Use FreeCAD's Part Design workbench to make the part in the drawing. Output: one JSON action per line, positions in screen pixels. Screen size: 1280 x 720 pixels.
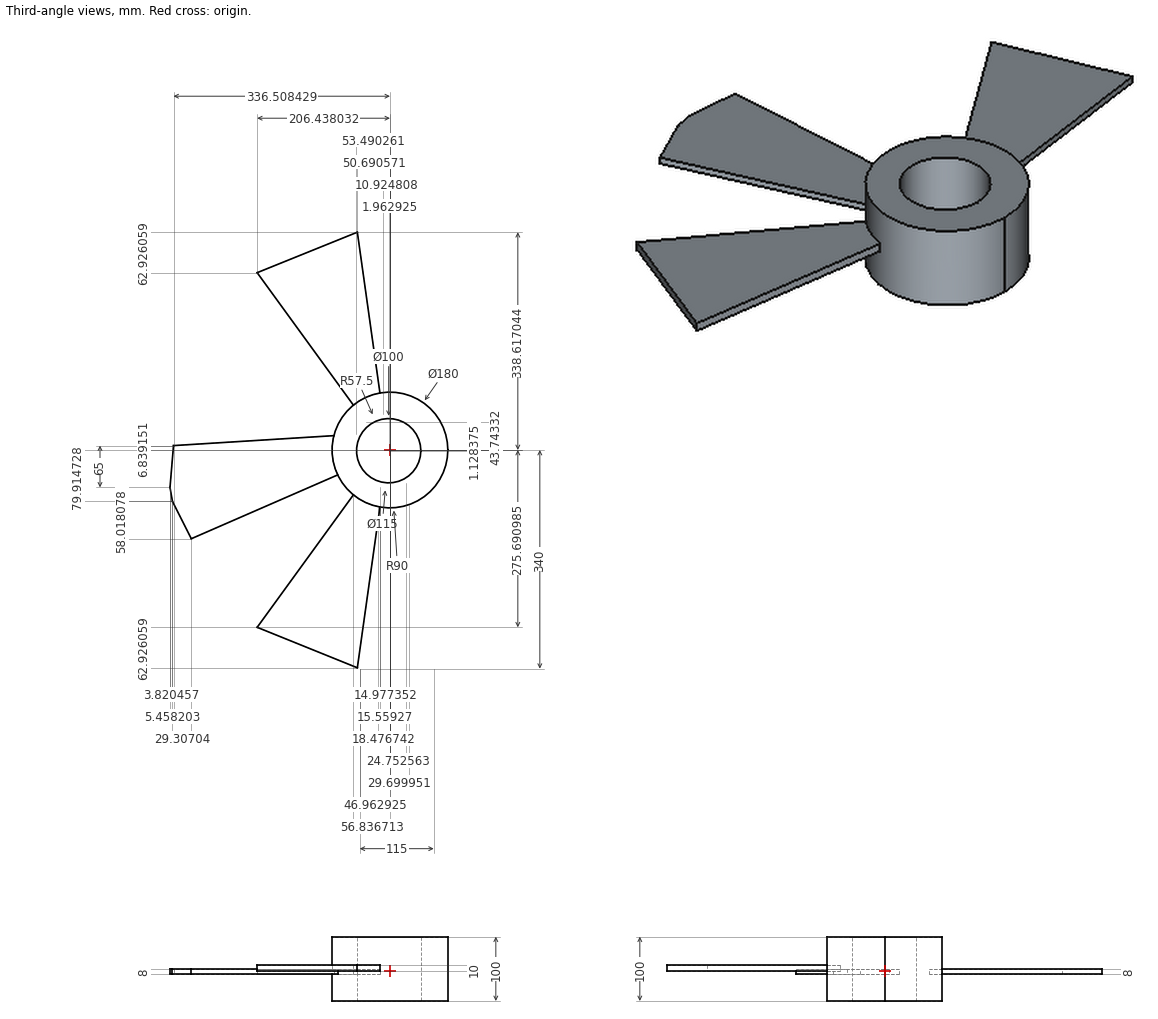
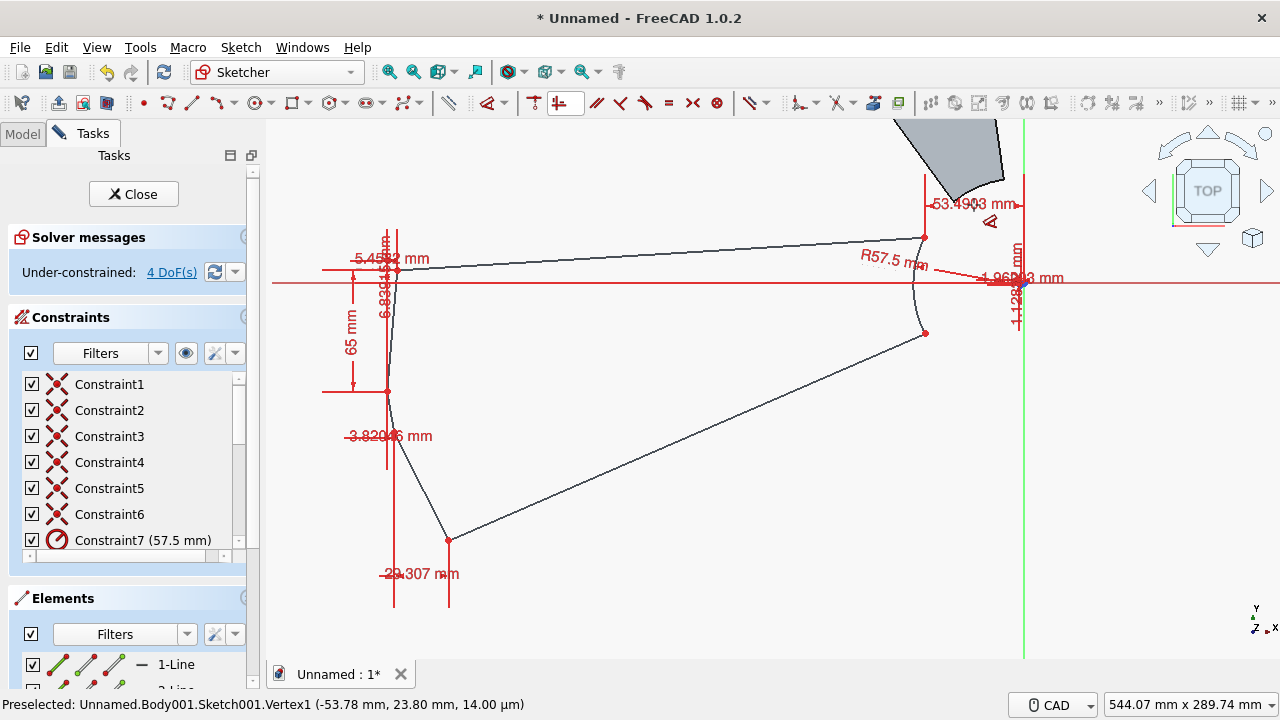
{"action": "left_click", "coordinate": [394, 433]}
{"action": "left_click", "coordinate": [1058, 358]}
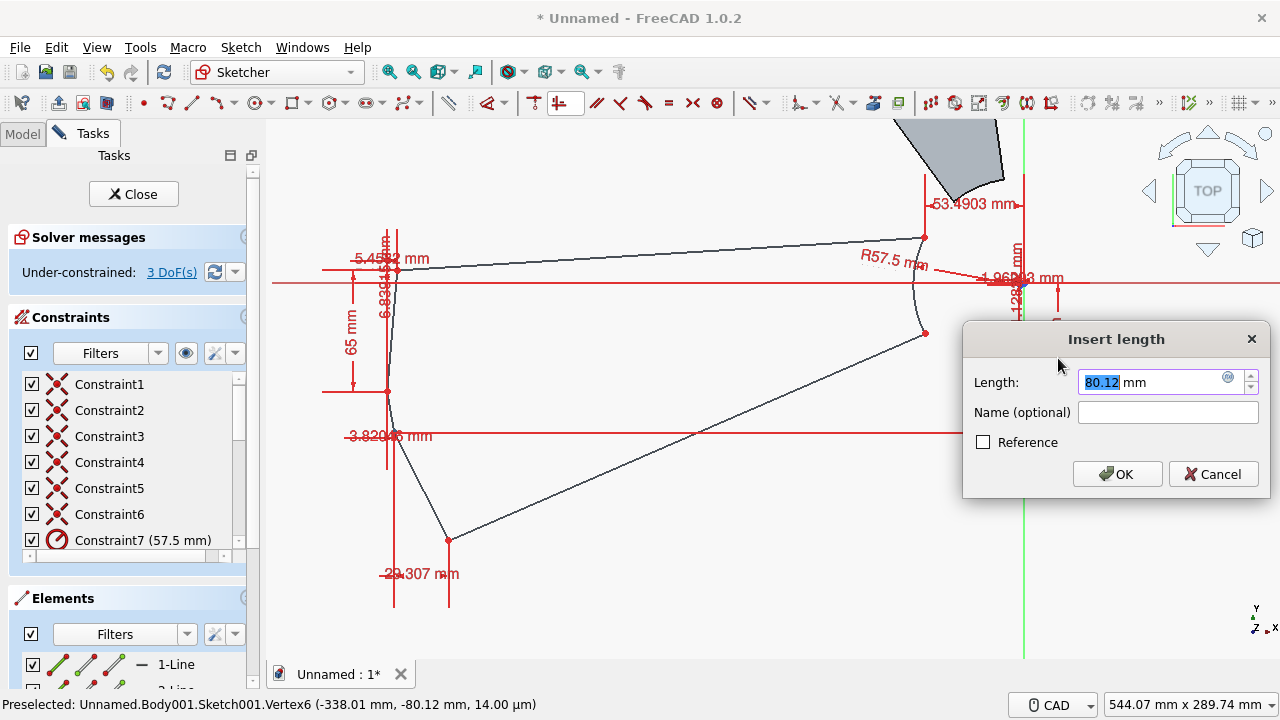
{"action": "type", "text": "79.914728"}
{"action": "key", "text": "Return"}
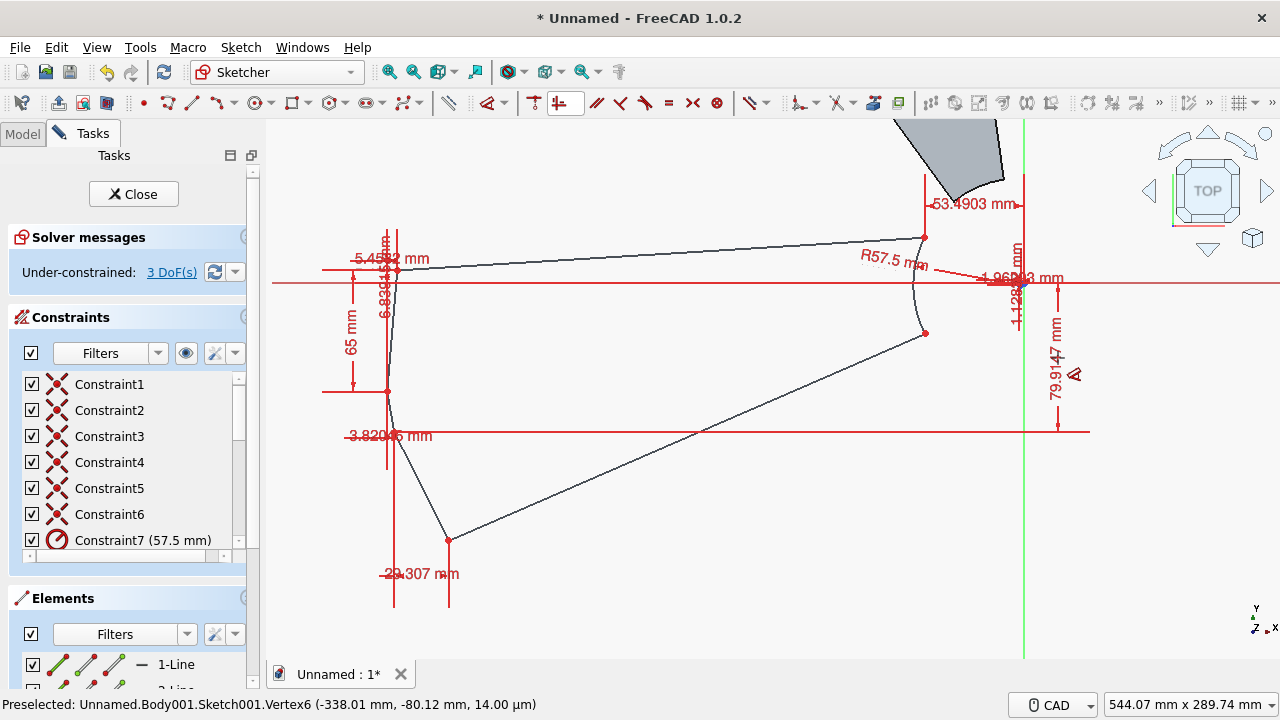
{"action": "left_click", "coordinate": [925, 334]}
{"action": "left_click", "coordinate": [975, 249]}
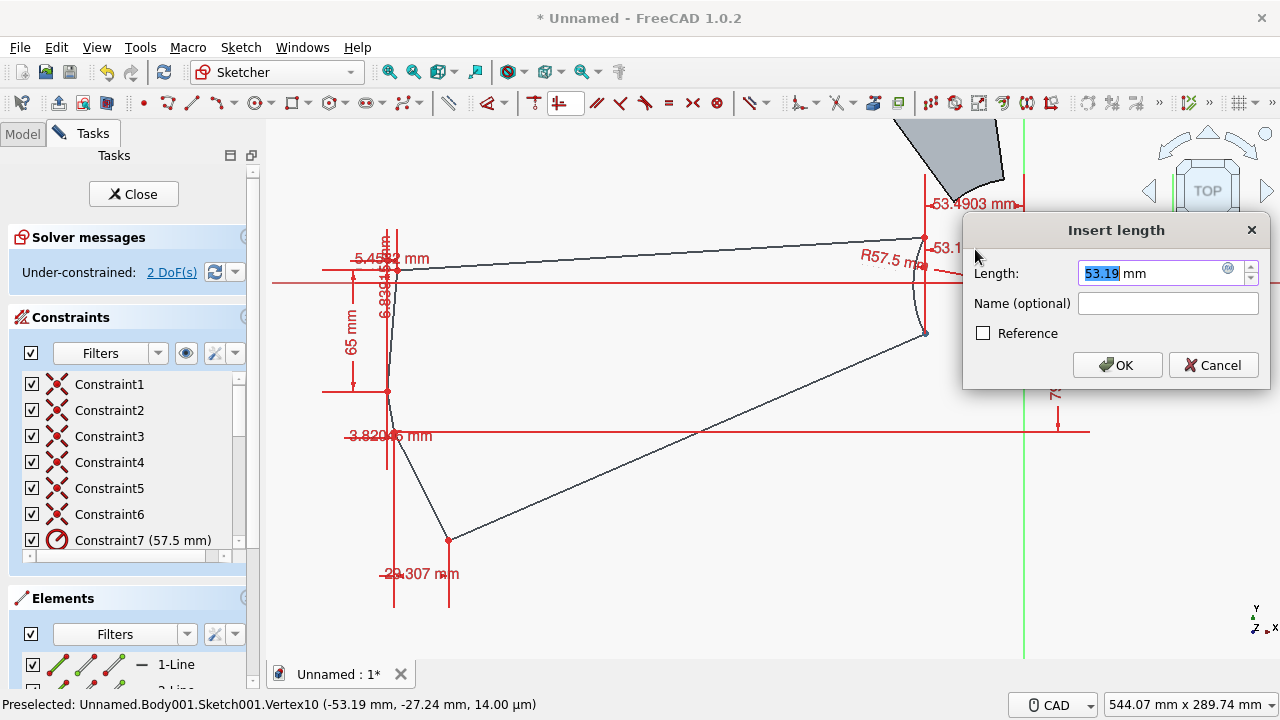
{"action": "type", "text": "53.490261"}
{"action": "key", "text": "Return"}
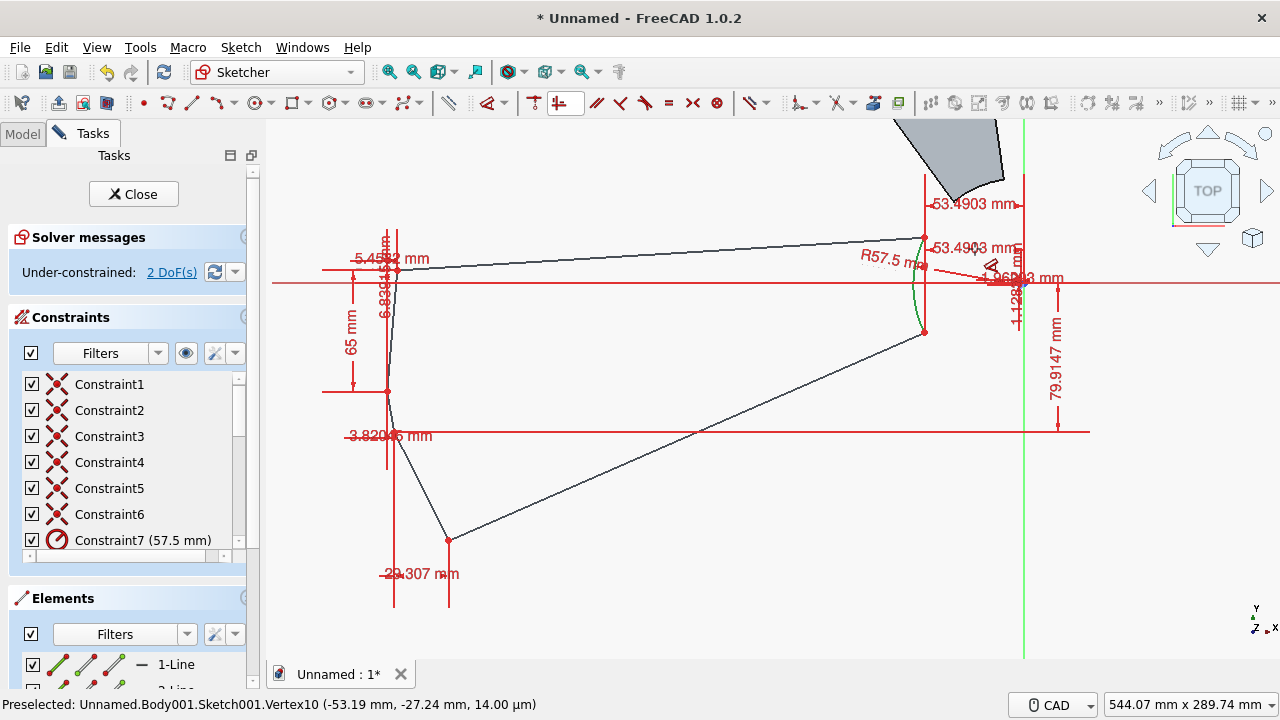
{"action": "left_click", "coordinate": [411, 465]}
{"action": "left_click", "coordinate": [360, 487]}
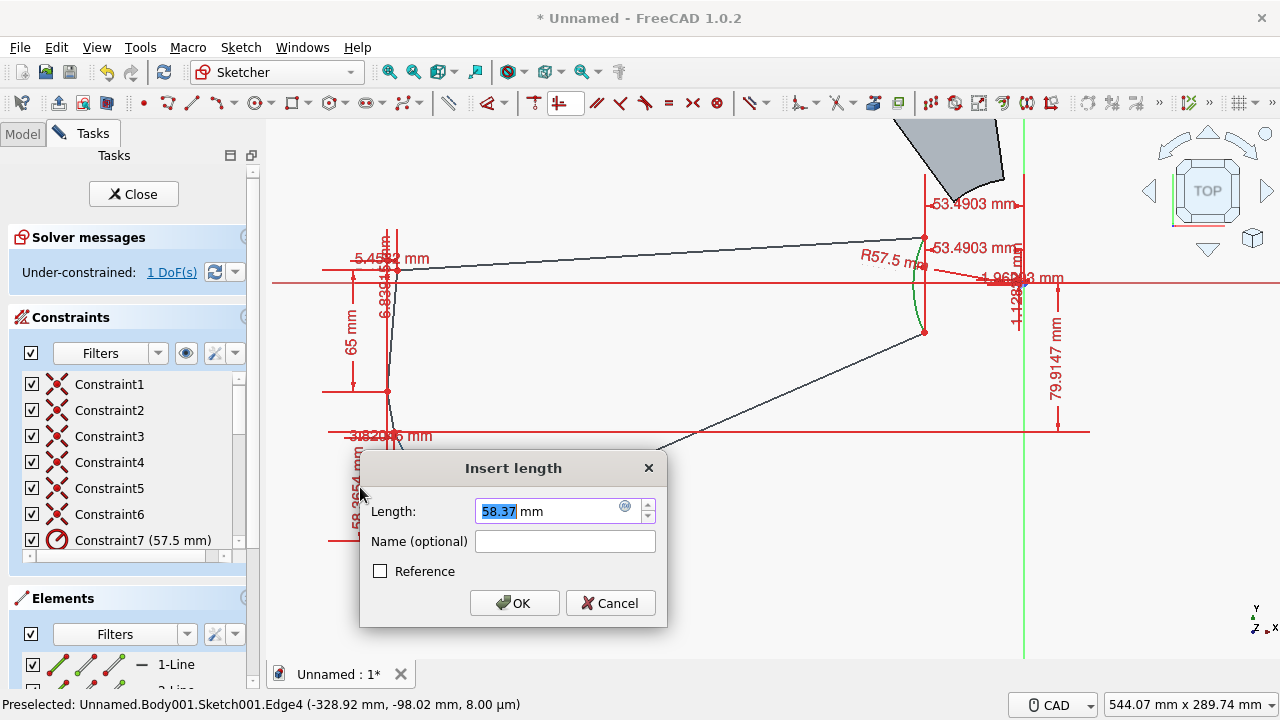
{"action": "type", "text": "58.018078"}
{"action": "key", "text": "Return"}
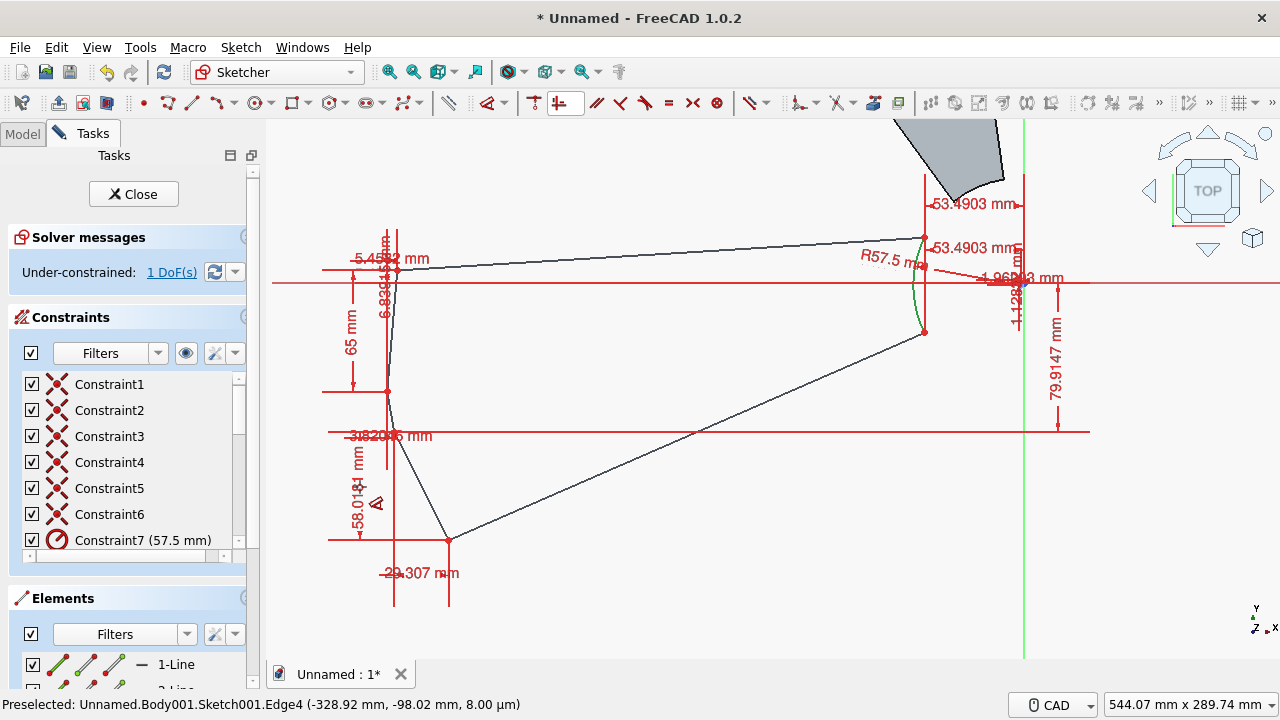
{"action": "left_click", "coordinate": [397, 270]}
{"action": "left_click", "coordinate": [711, 236]}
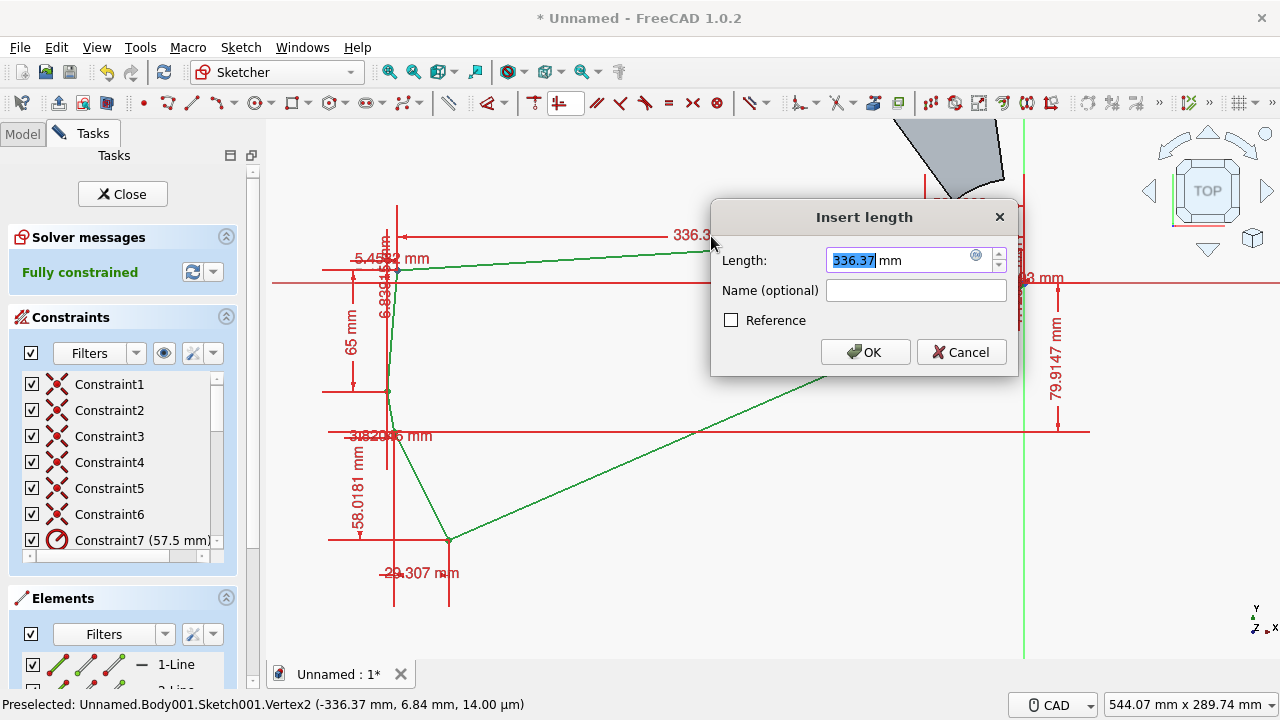
{"action": "type", "text": "336.508429"}
{"action": "key", "text": "Return"}
{"action": "key", "text": "Escape"}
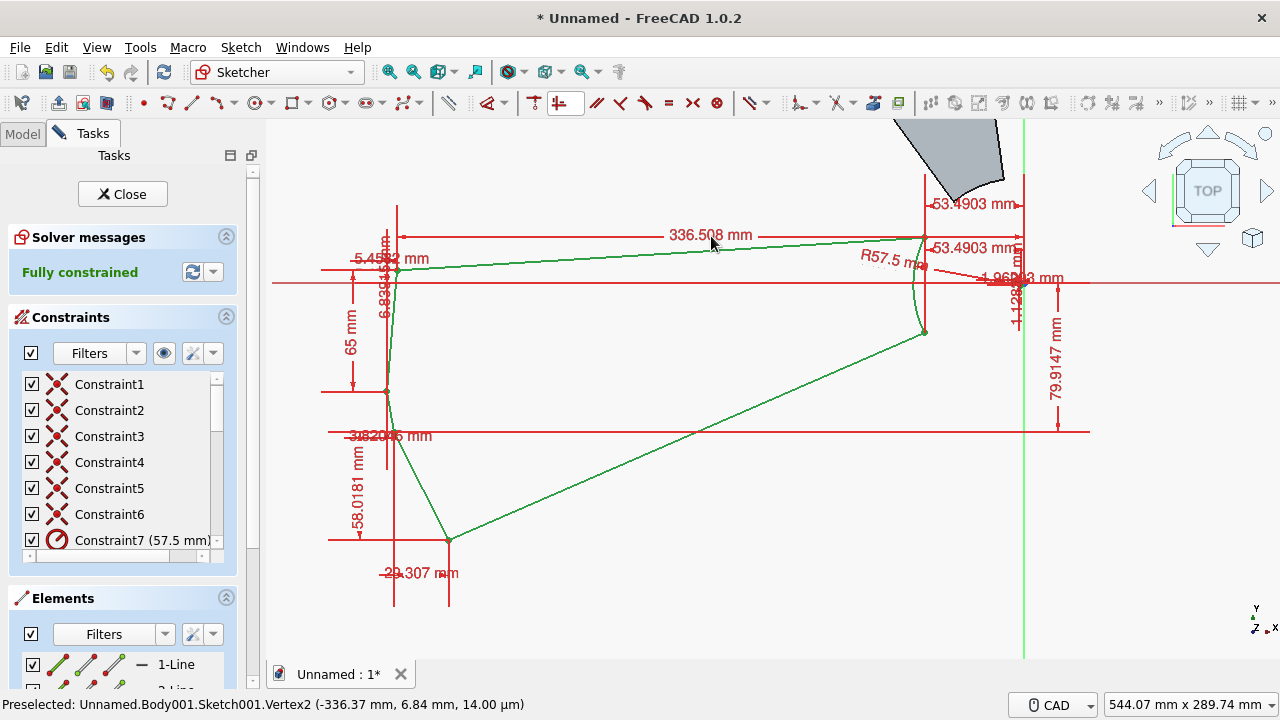
{"action": "left_click", "coordinate": [123, 194]}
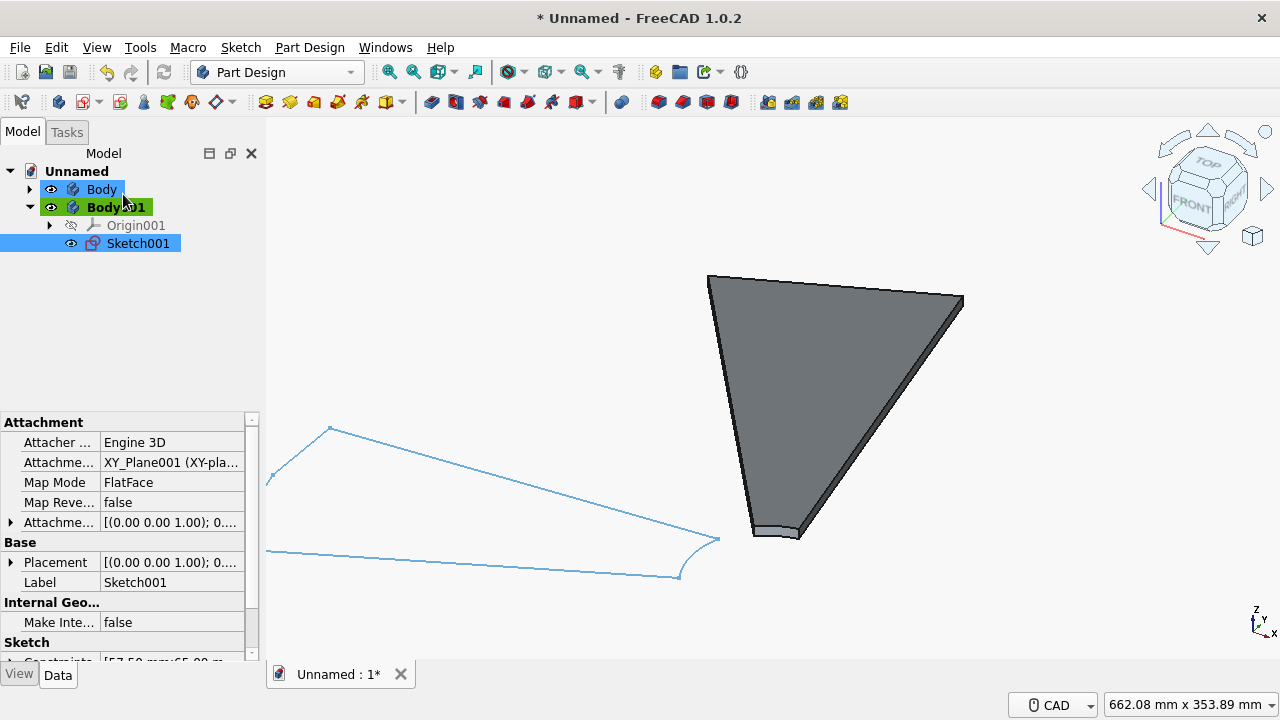
{"action": "left_click", "coordinate": [266, 102]}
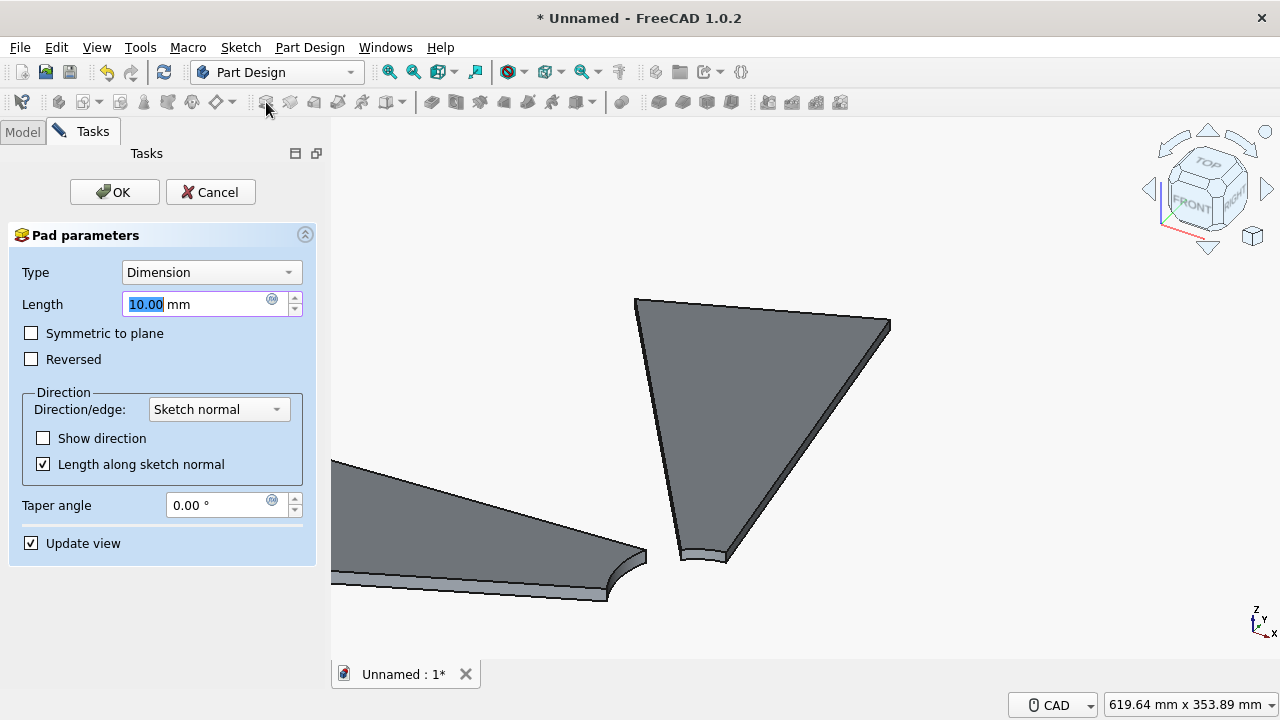
{"action": "type", "text": "8"}
{"action": "key", "text": "Tab"}